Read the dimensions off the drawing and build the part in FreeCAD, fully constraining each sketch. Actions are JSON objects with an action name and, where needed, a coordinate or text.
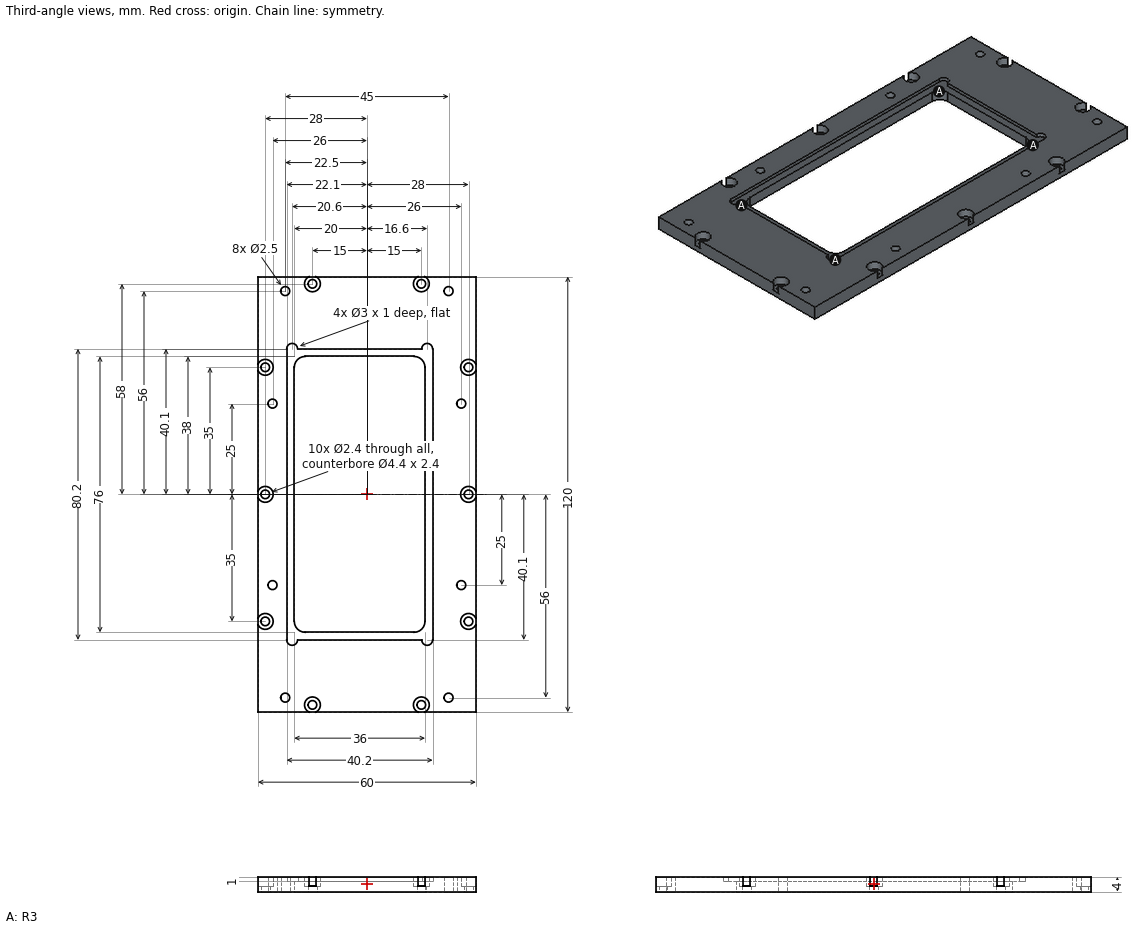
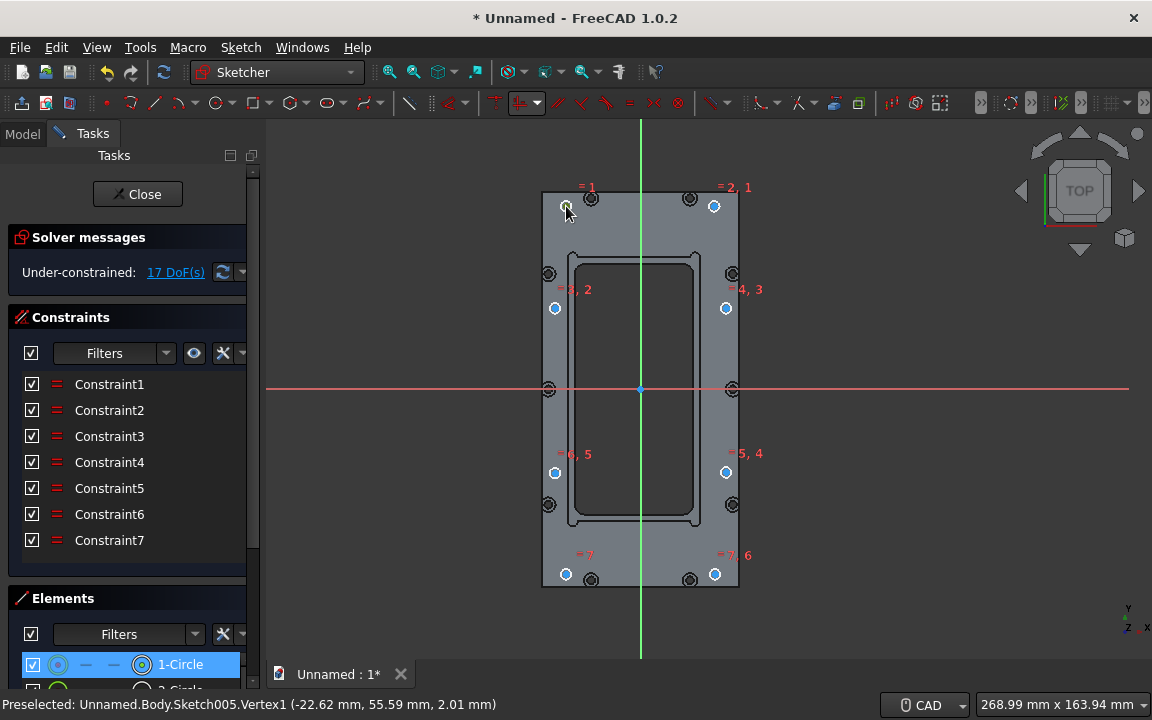
{"action": "left_click", "coordinate": [714, 206]}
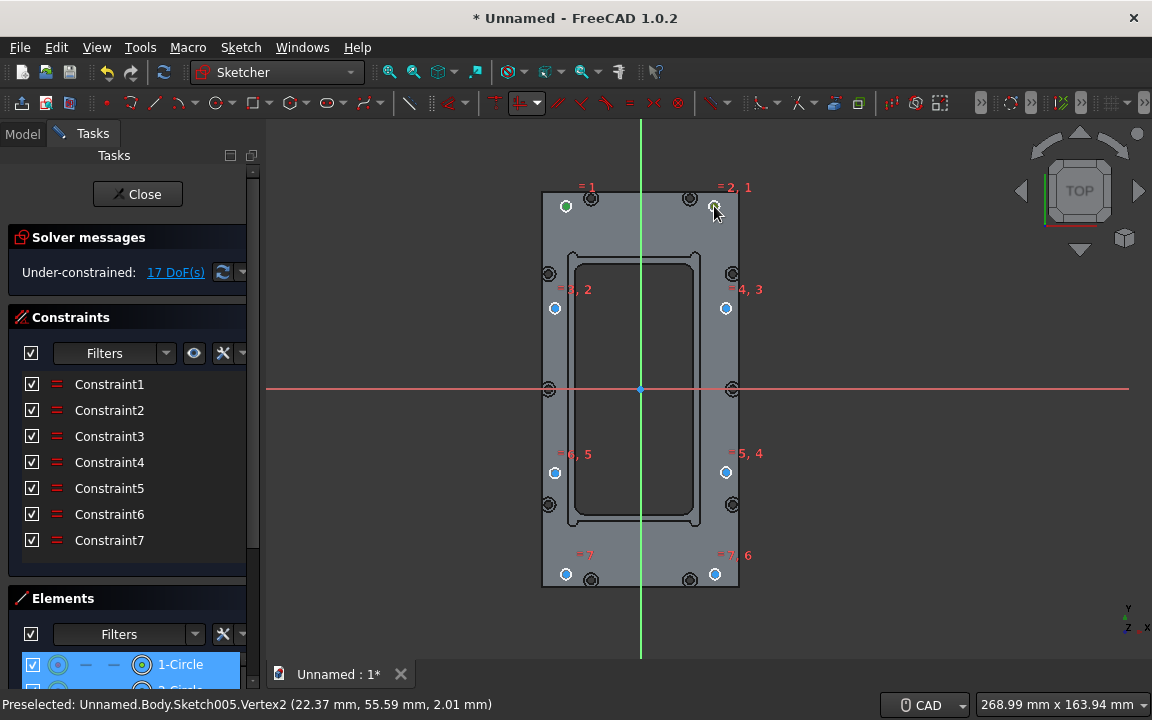
{"action": "left_click", "coordinate": [540, 104]}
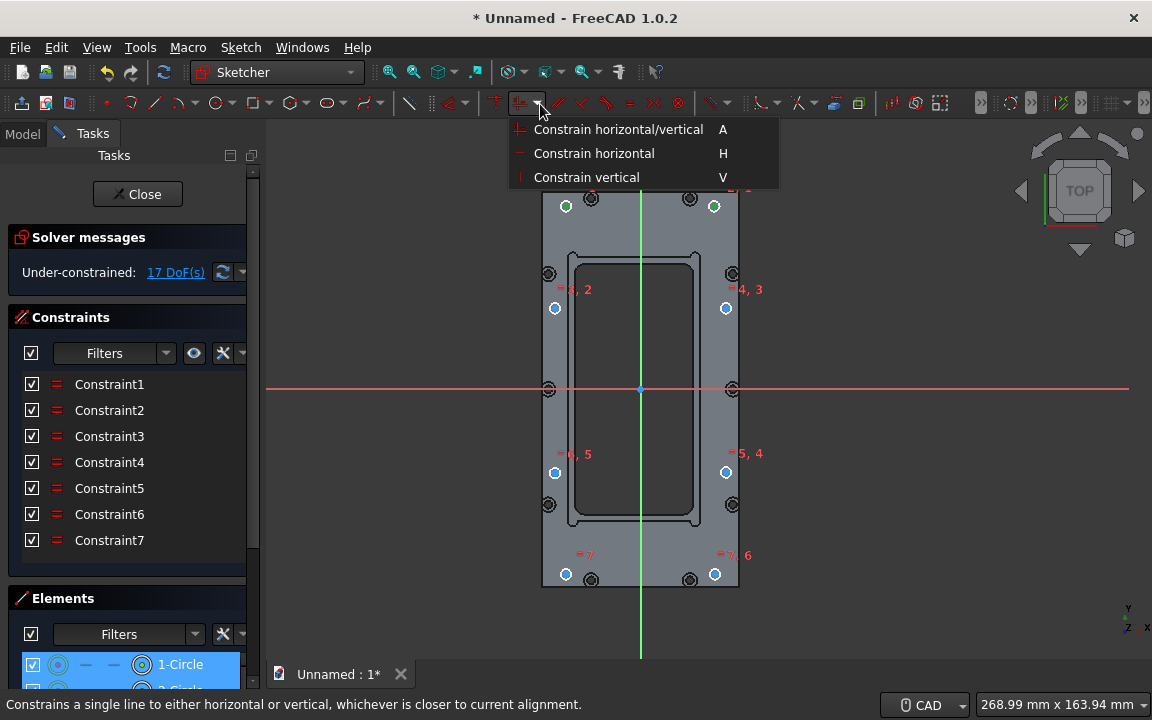
{"action": "left_click", "coordinate": [644, 153]}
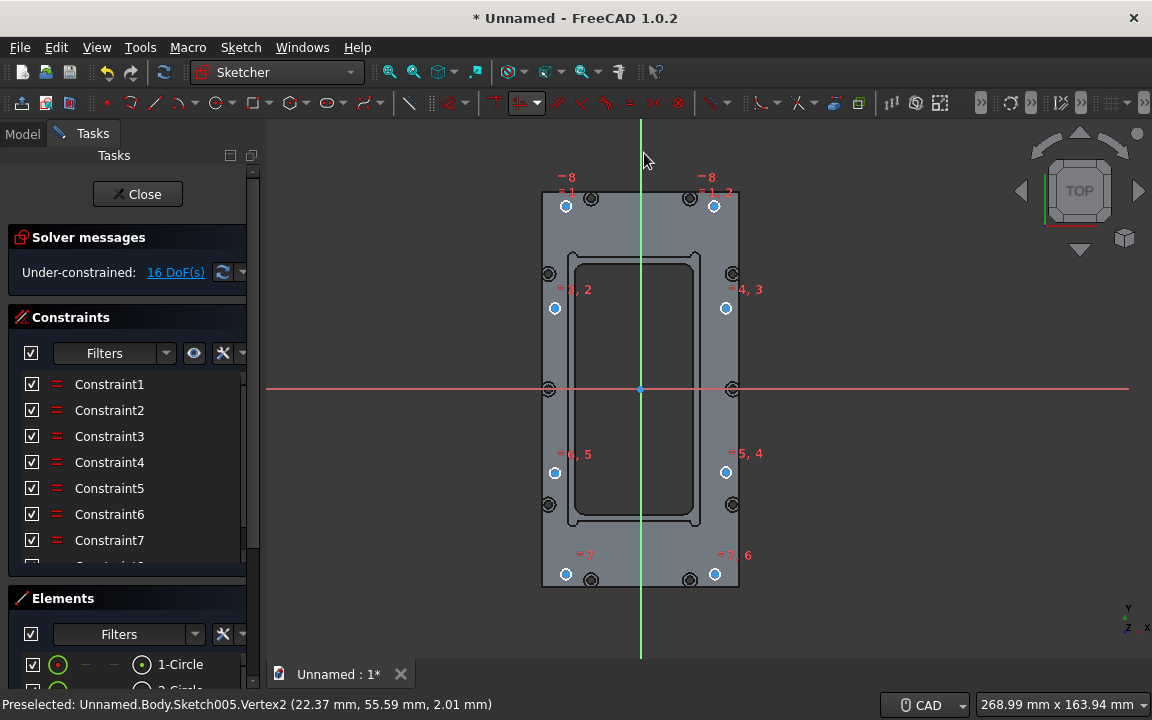
{"action": "left_click", "coordinate": [555, 308]}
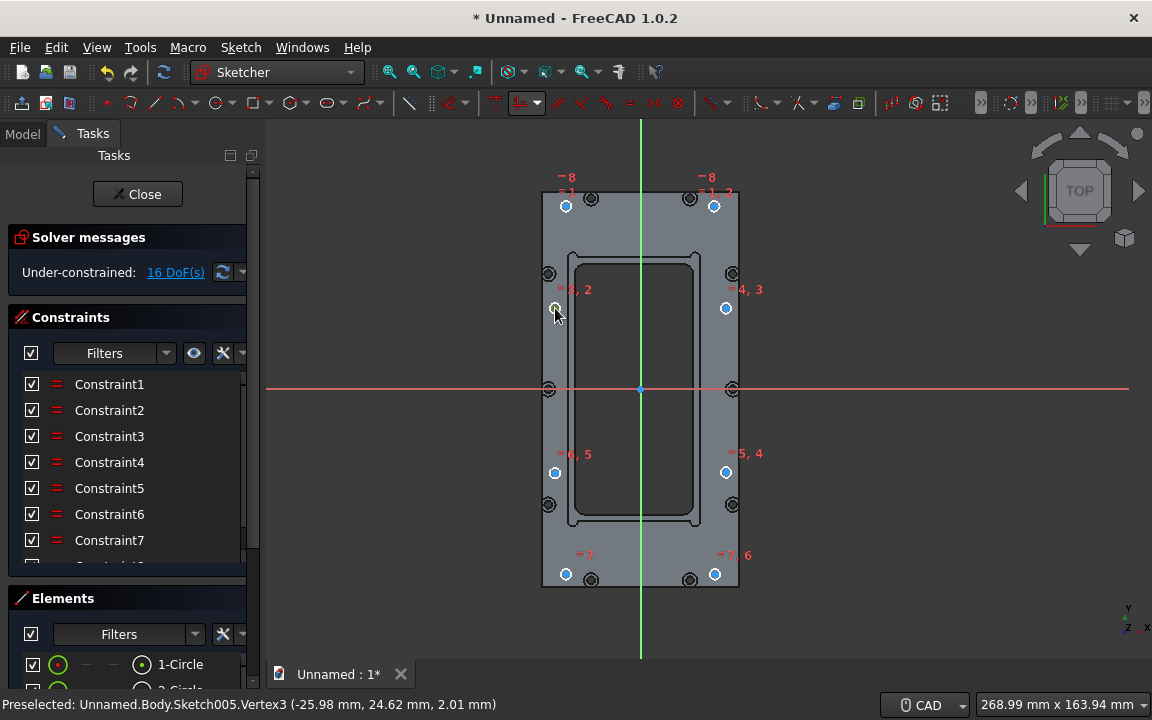
{"action": "left_click", "coordinate": [726, 308]}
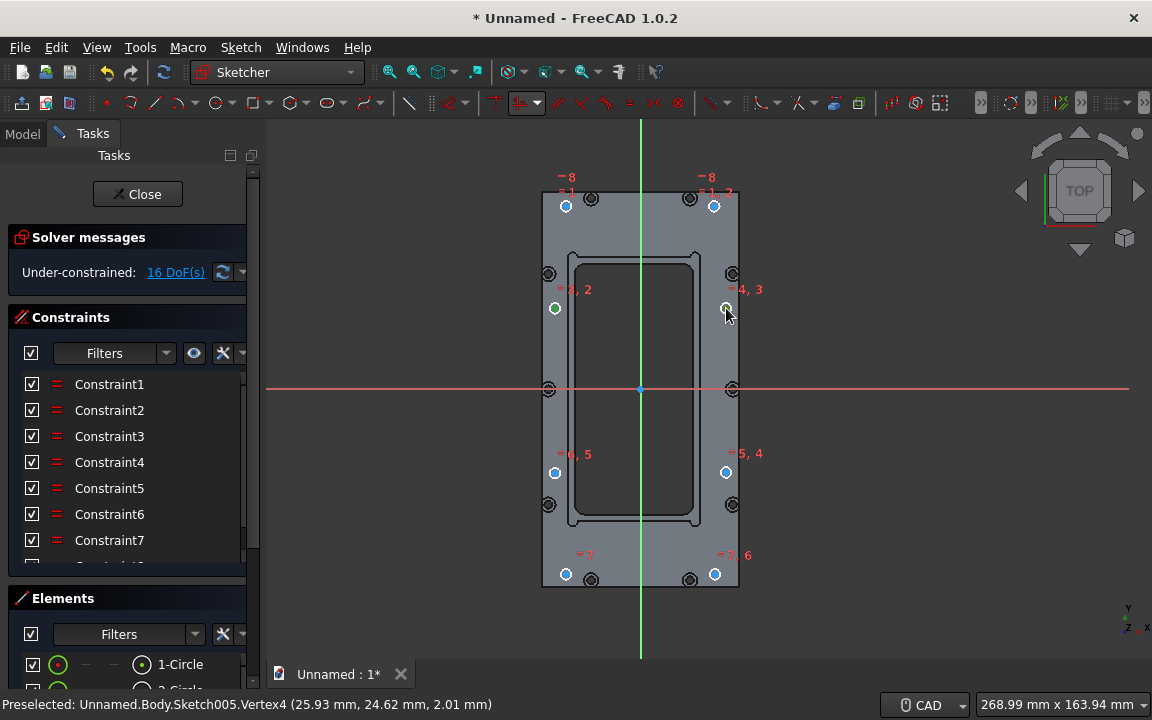
{"action": "key", "text": "h"}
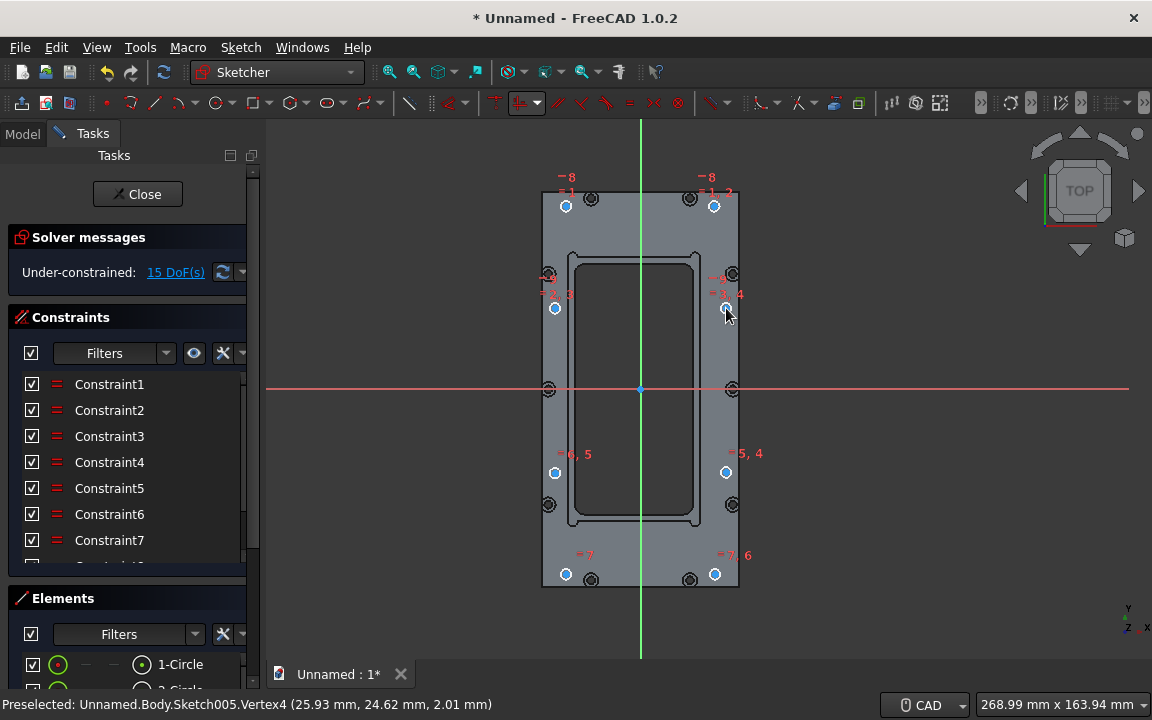
{"action": "left_click", "coordinate": [726, 308]}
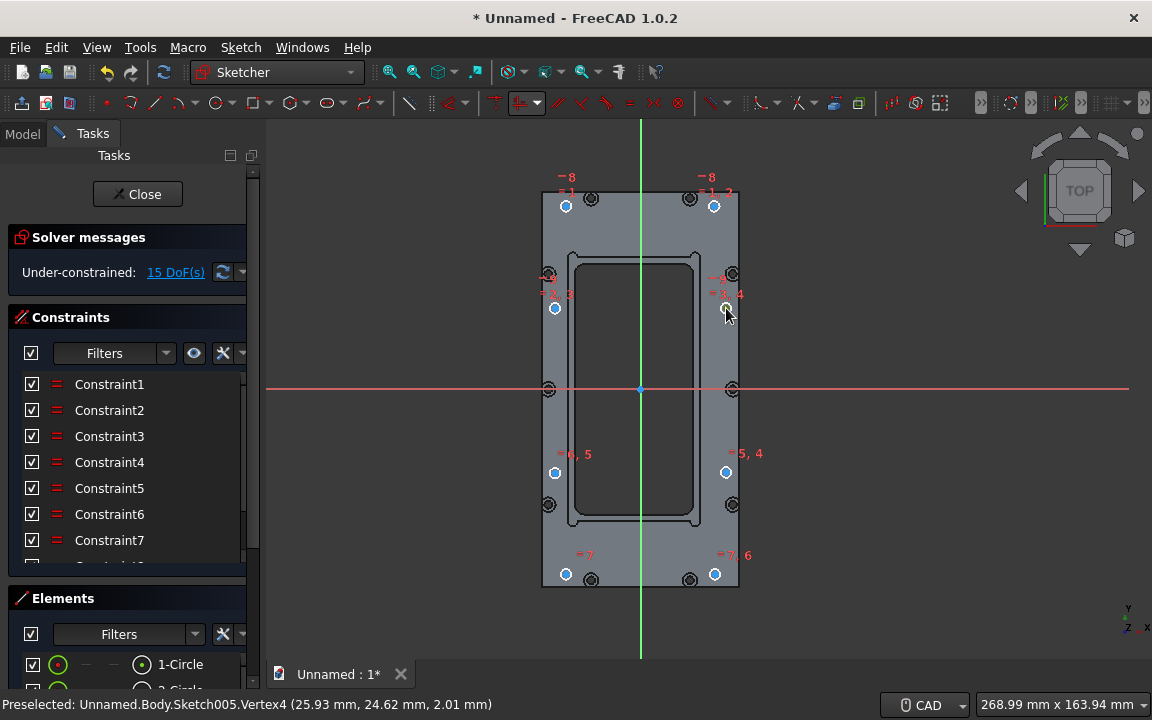
{"action": "left_click", "coordinate": [726, 472]}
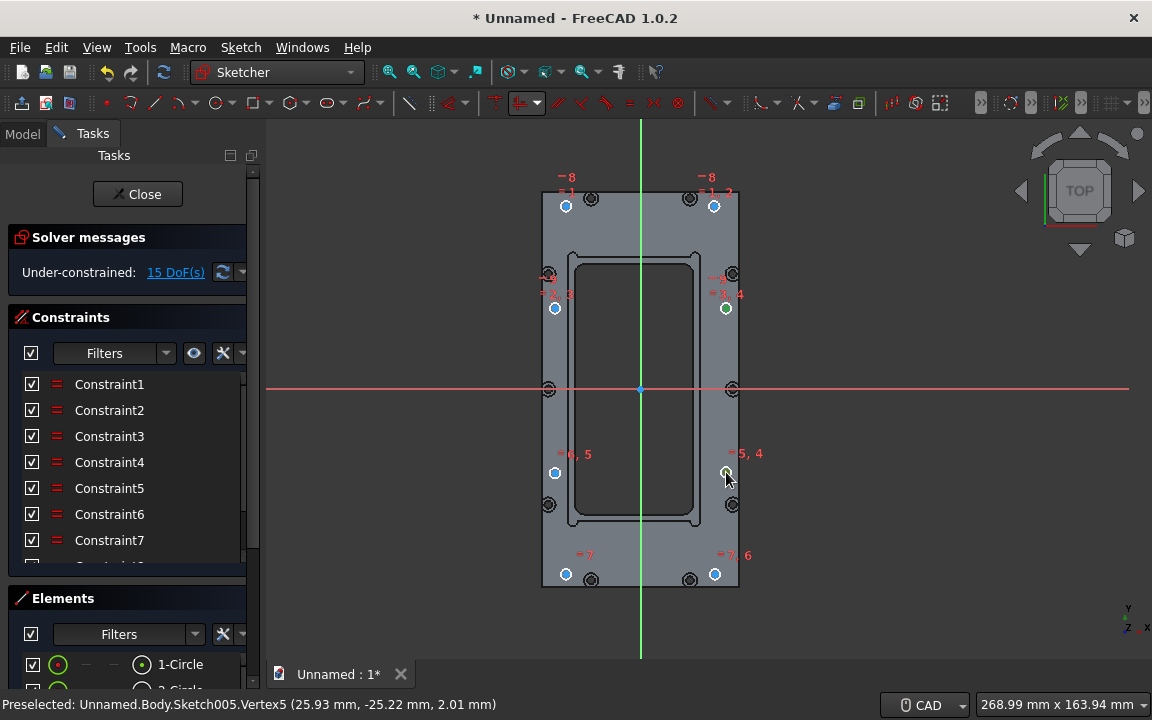
{"action": "key", "text": "v"}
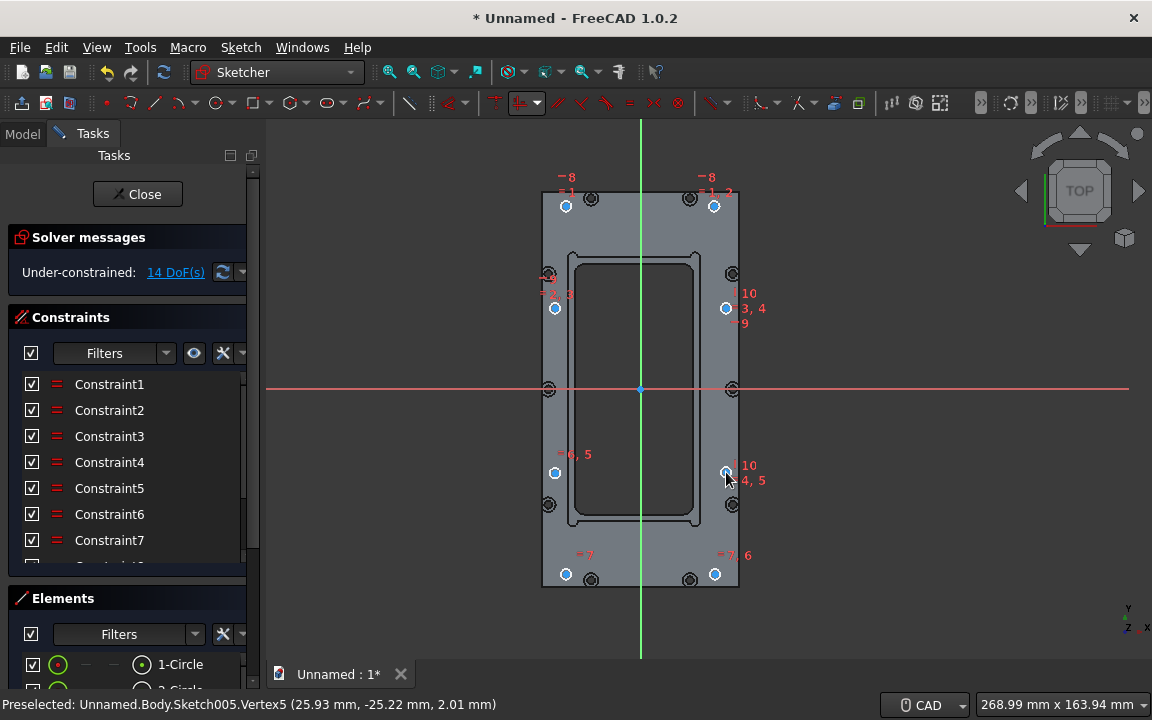
{"action": "left_click", "coordinate": [555, 308]}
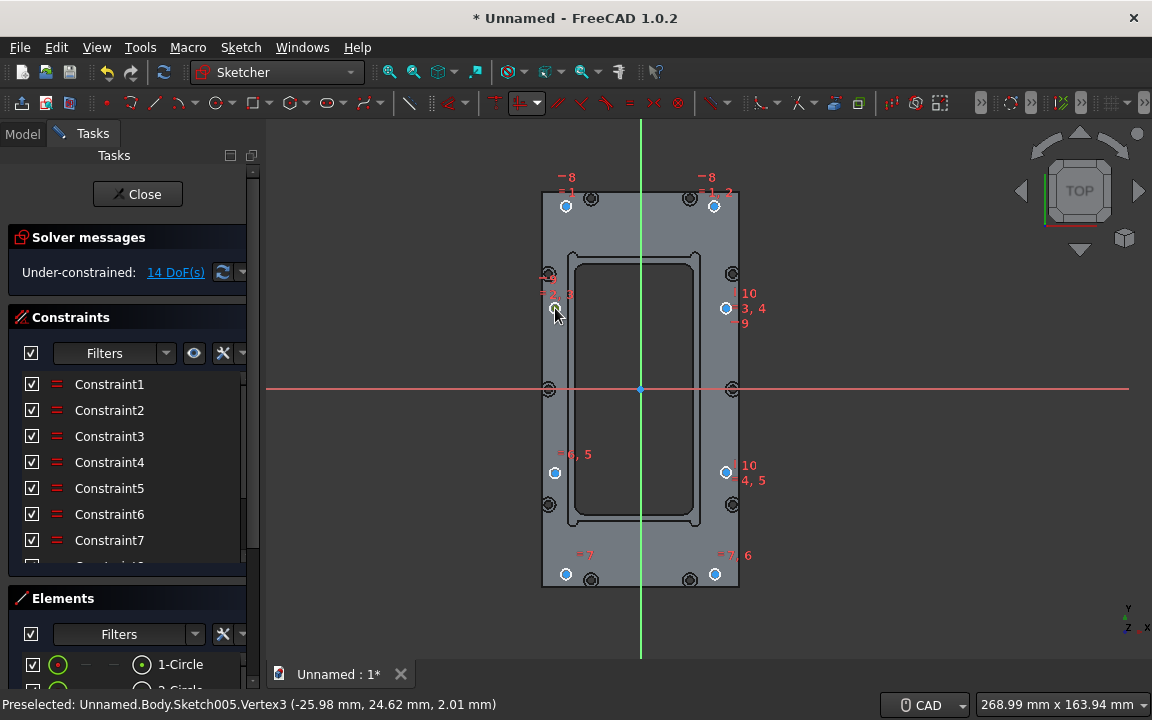
{"action": "left_click", "coordinate": [555, 473]}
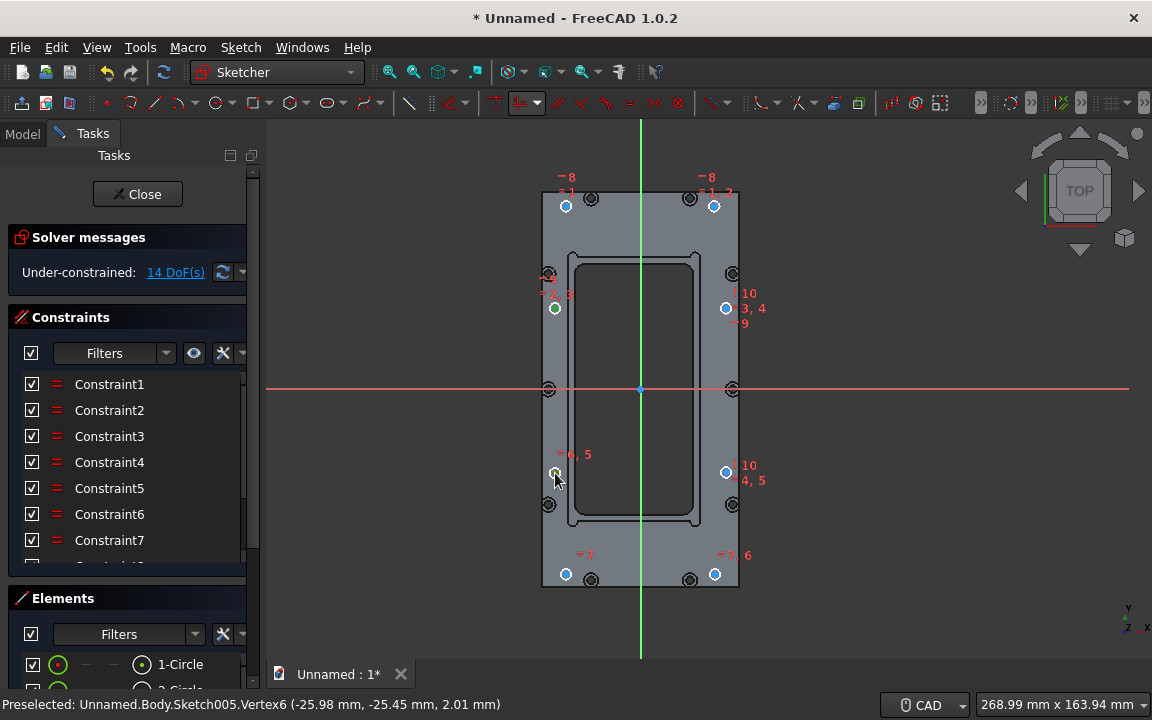
{"action": "key", "text": "v"}